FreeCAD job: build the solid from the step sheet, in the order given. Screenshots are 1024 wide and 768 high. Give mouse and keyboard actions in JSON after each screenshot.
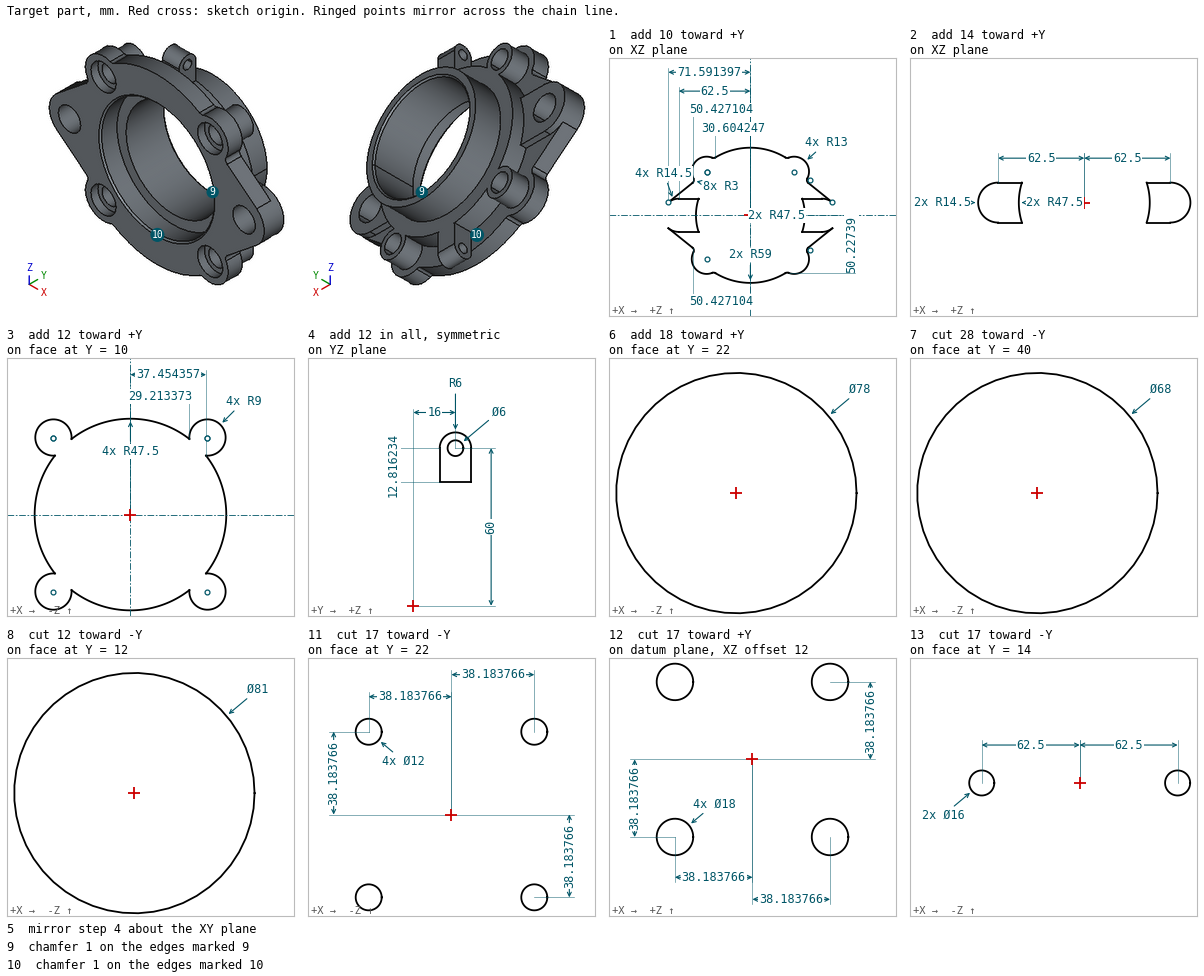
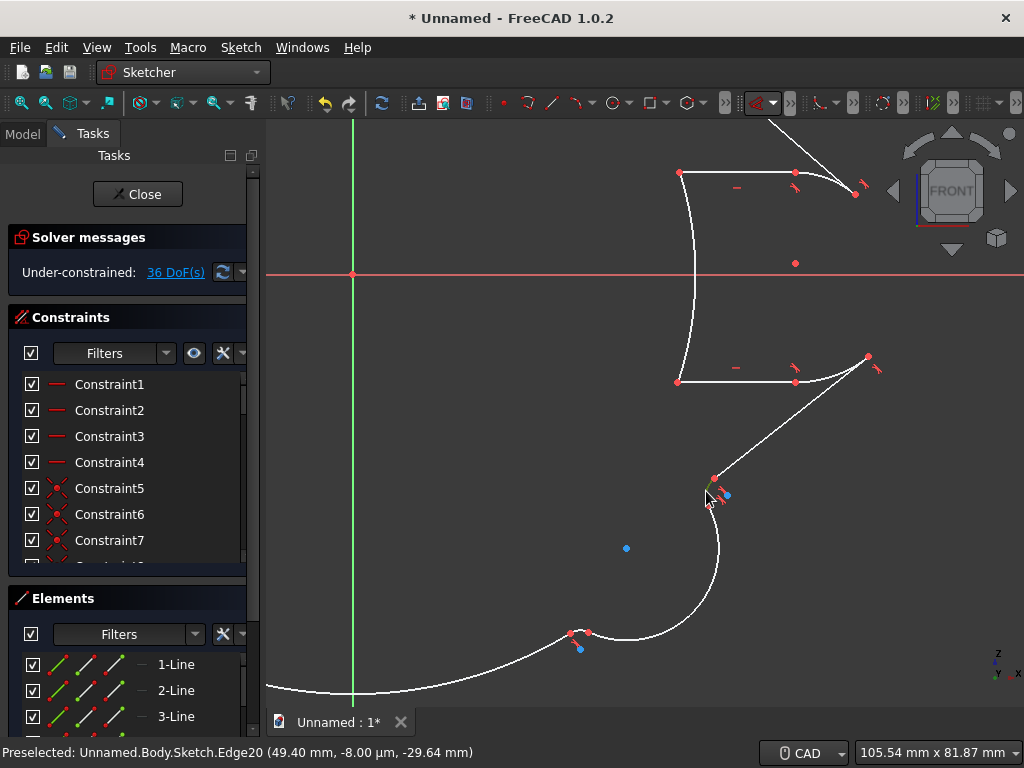
{"action": "scroll", "coordinate": [580, 630], "scroll_direction": "up", "scroll_amount": 3}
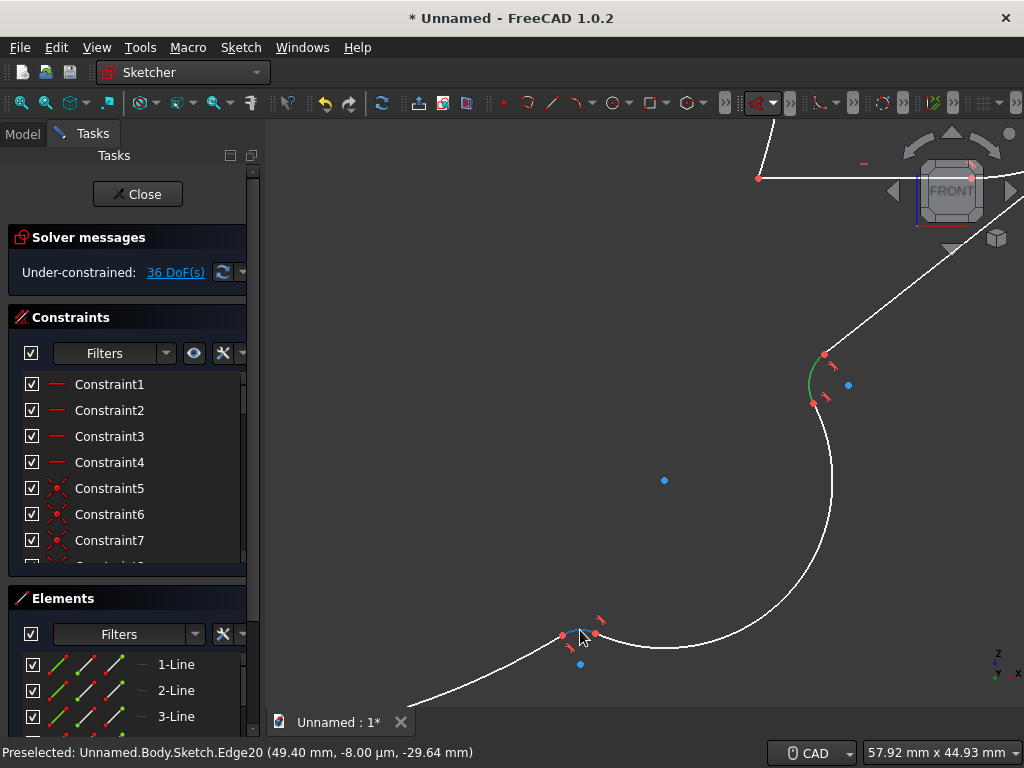
{"action": "left_click", "coordinate": [579, 630]}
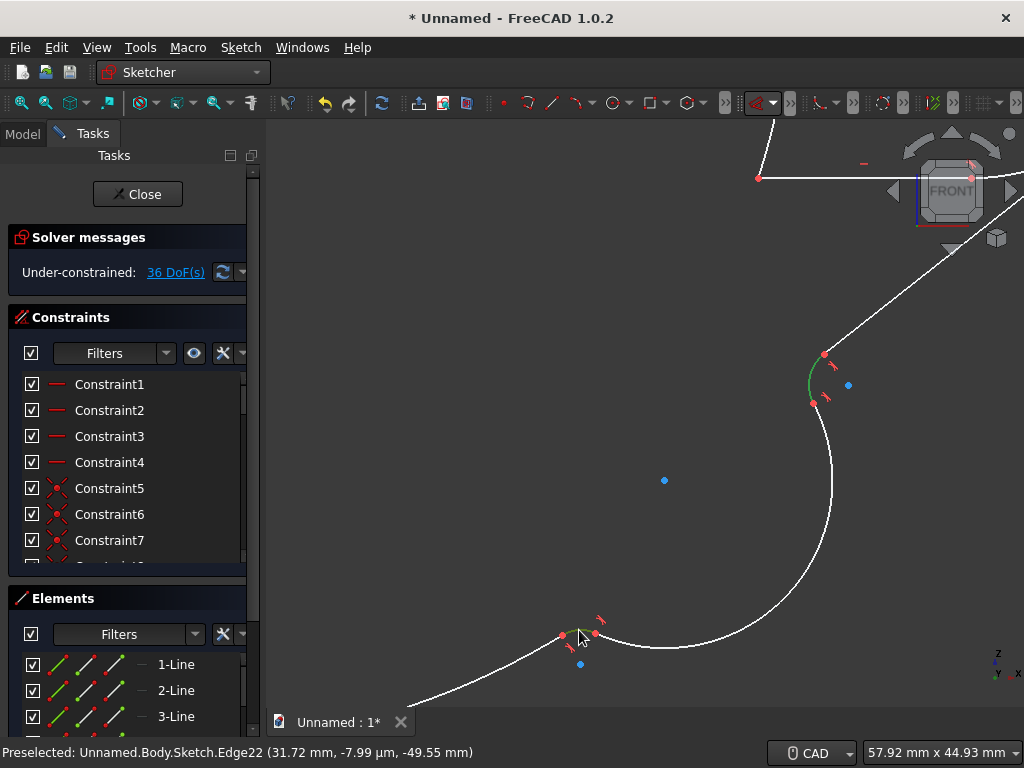
{"action": "scroll", "coordinate": [680, 522], "scroll_direction": "down", "scroll_amount": 8}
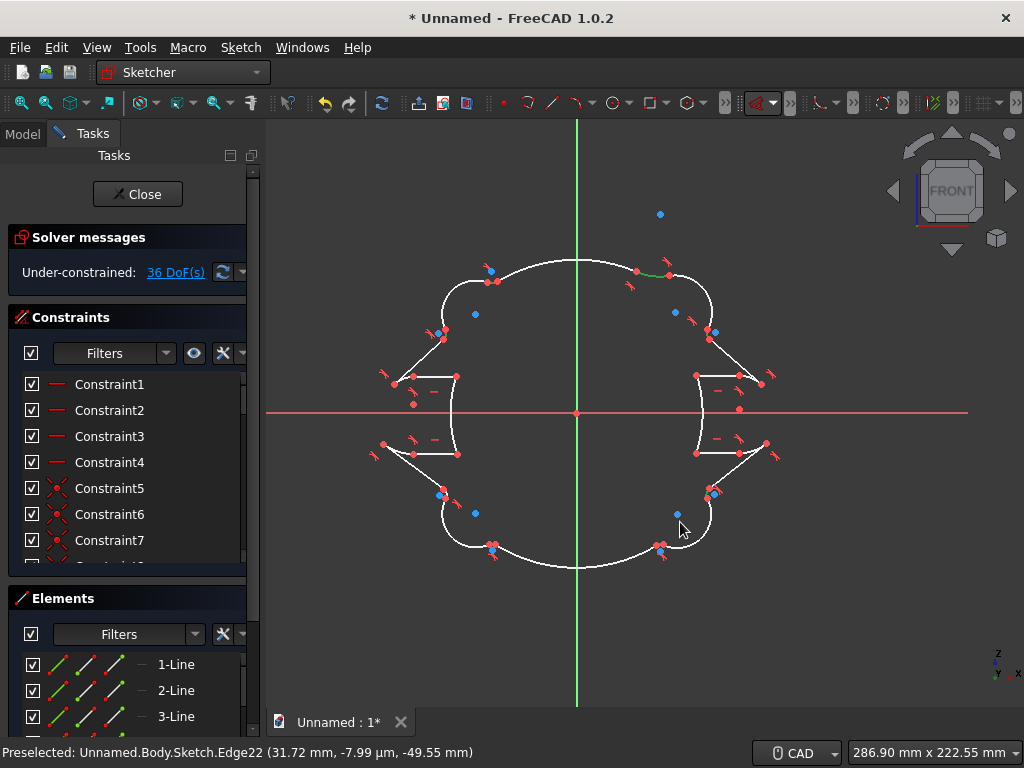
{"action": "scroll", "coordinate": [494, 544], "scroll_direction": "up", "scroll_amount": 10}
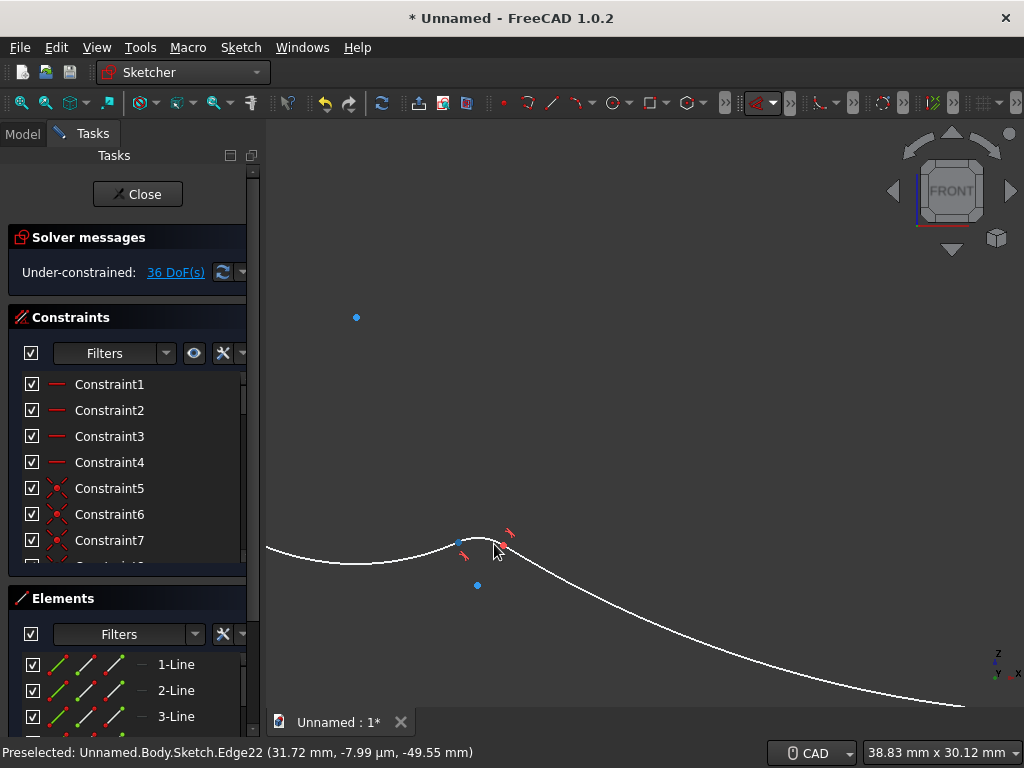
{"action": "left_click", "coordinate": [490, 540]}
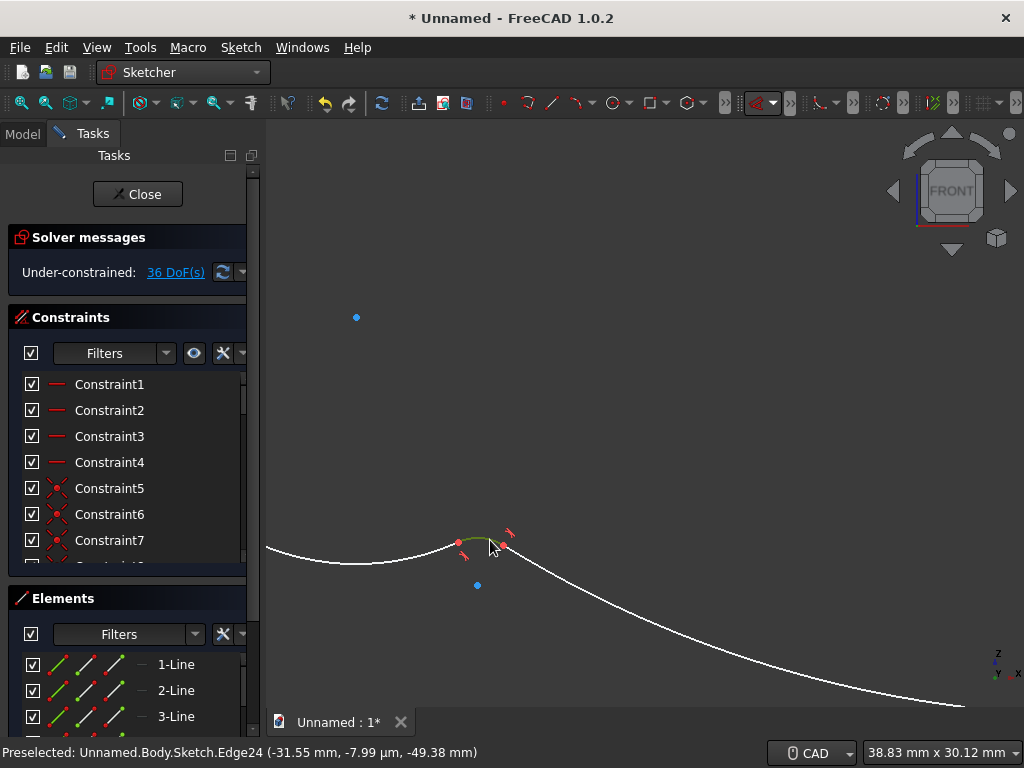
{"action": "scroll", "coordinate": [494, 544], "scroll_direction": "down", "scroll_amount": 10}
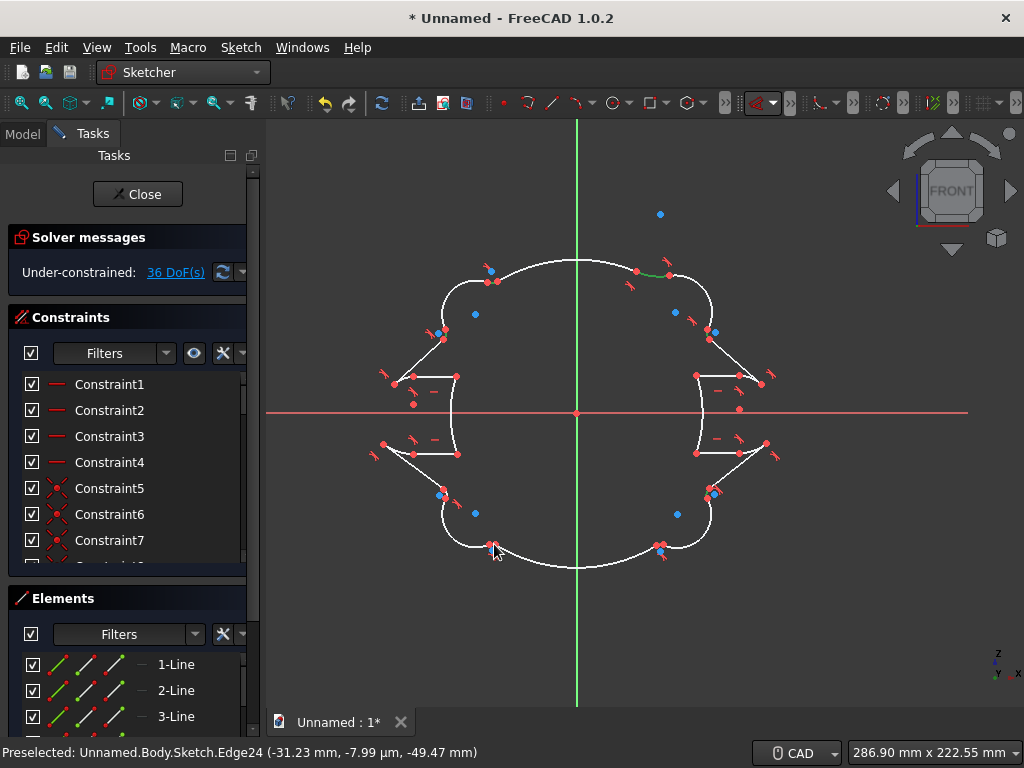
{"action": "scroll", "coordinate": [447, 496], "scroll_direction": "up", "scroll_amount": 8}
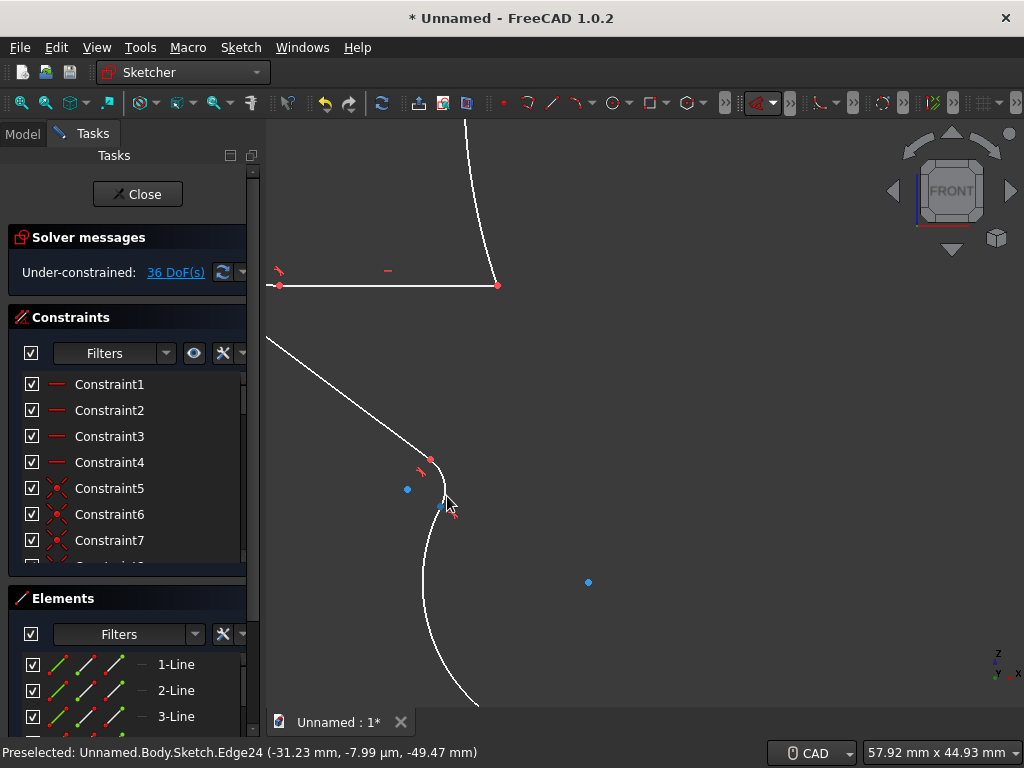
{"action": "left_click", "coordinate": [445, 492]}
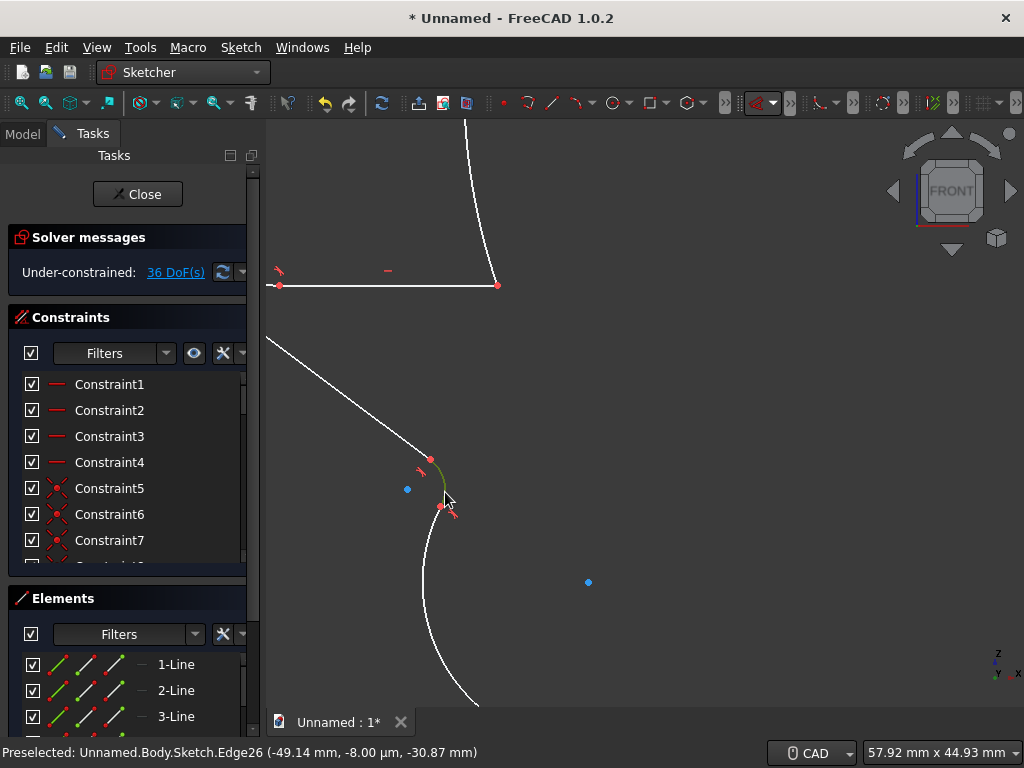
{"action": "key", "text": "e"}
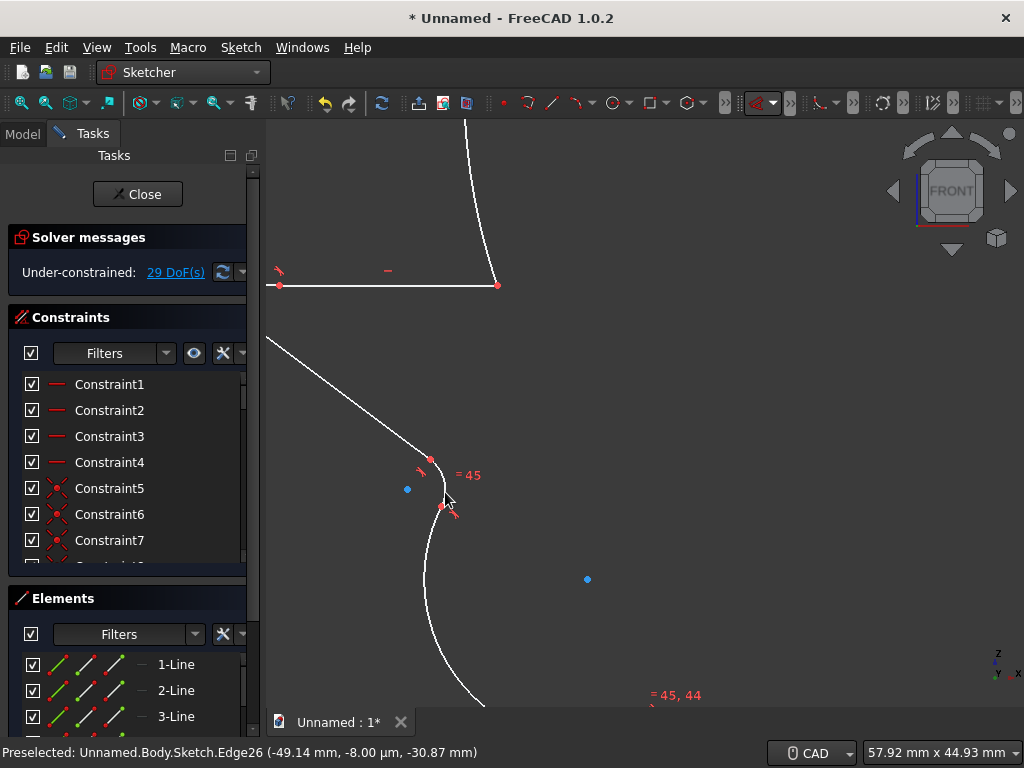
{"action": "scroll", "coordinate": [447, 496], "scroll_direction": "down", "scroll_amount": 8}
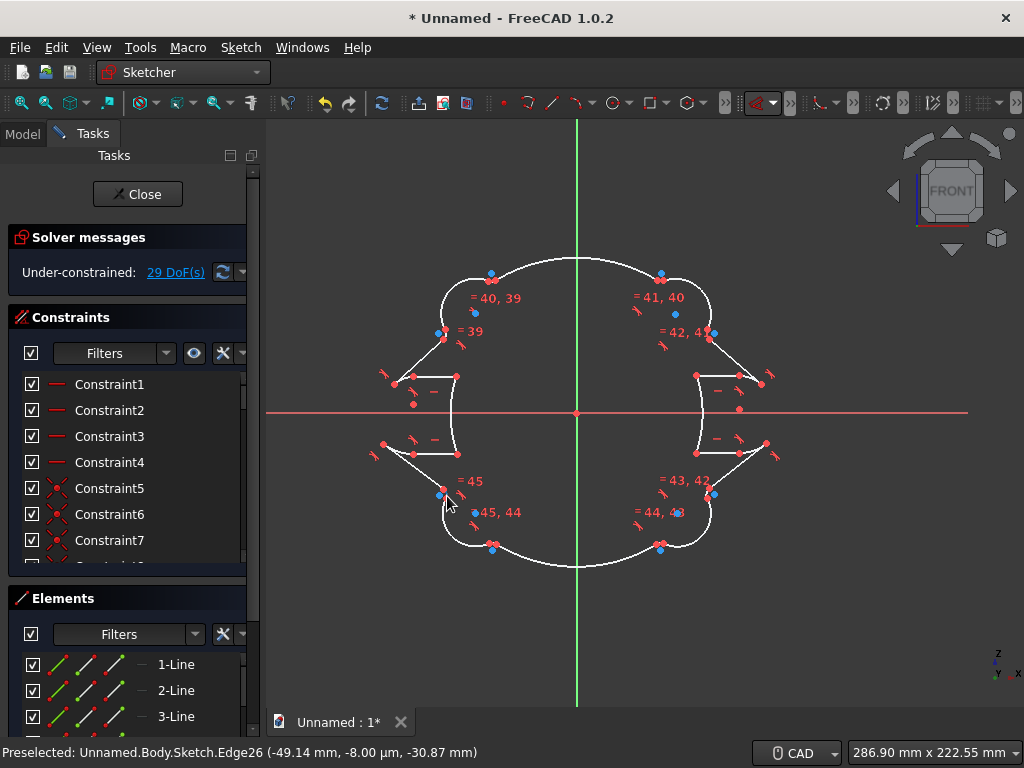
{"action": "left_click", "coordinate": [464, 281]}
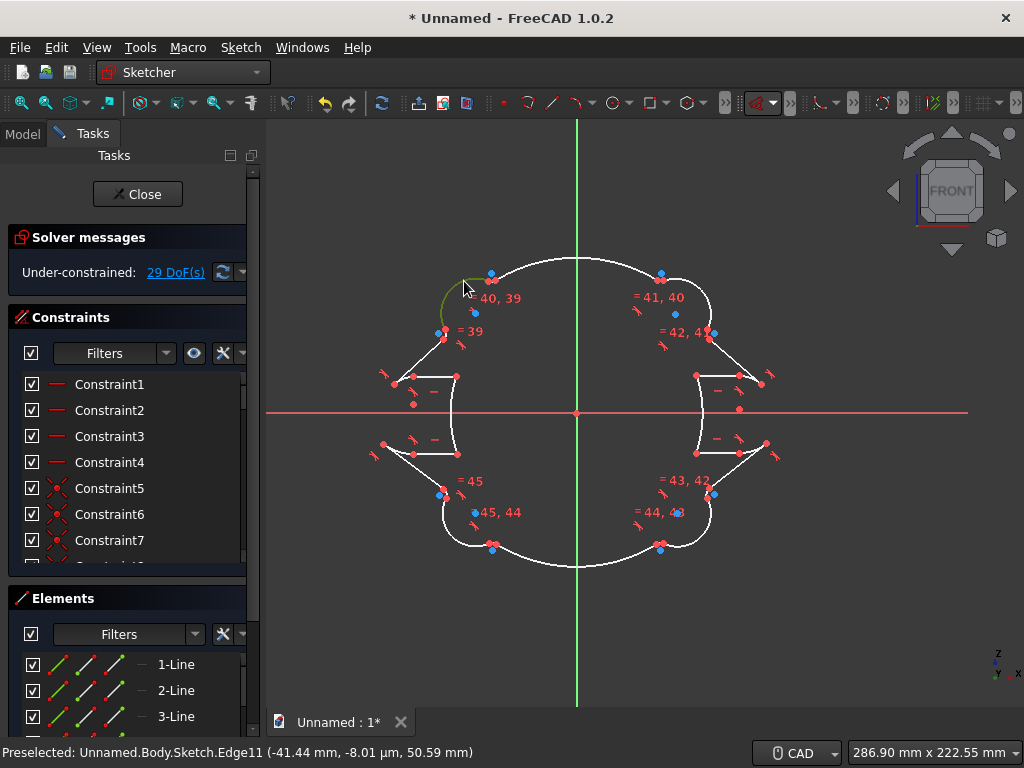
{"action": "left_click", "coordinate": [710, 305]}